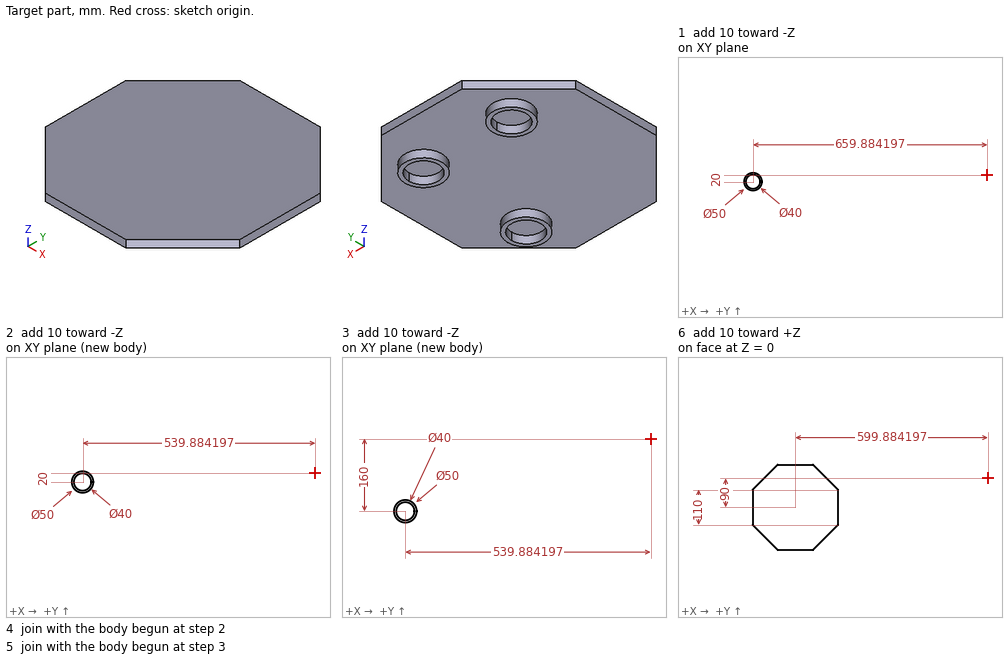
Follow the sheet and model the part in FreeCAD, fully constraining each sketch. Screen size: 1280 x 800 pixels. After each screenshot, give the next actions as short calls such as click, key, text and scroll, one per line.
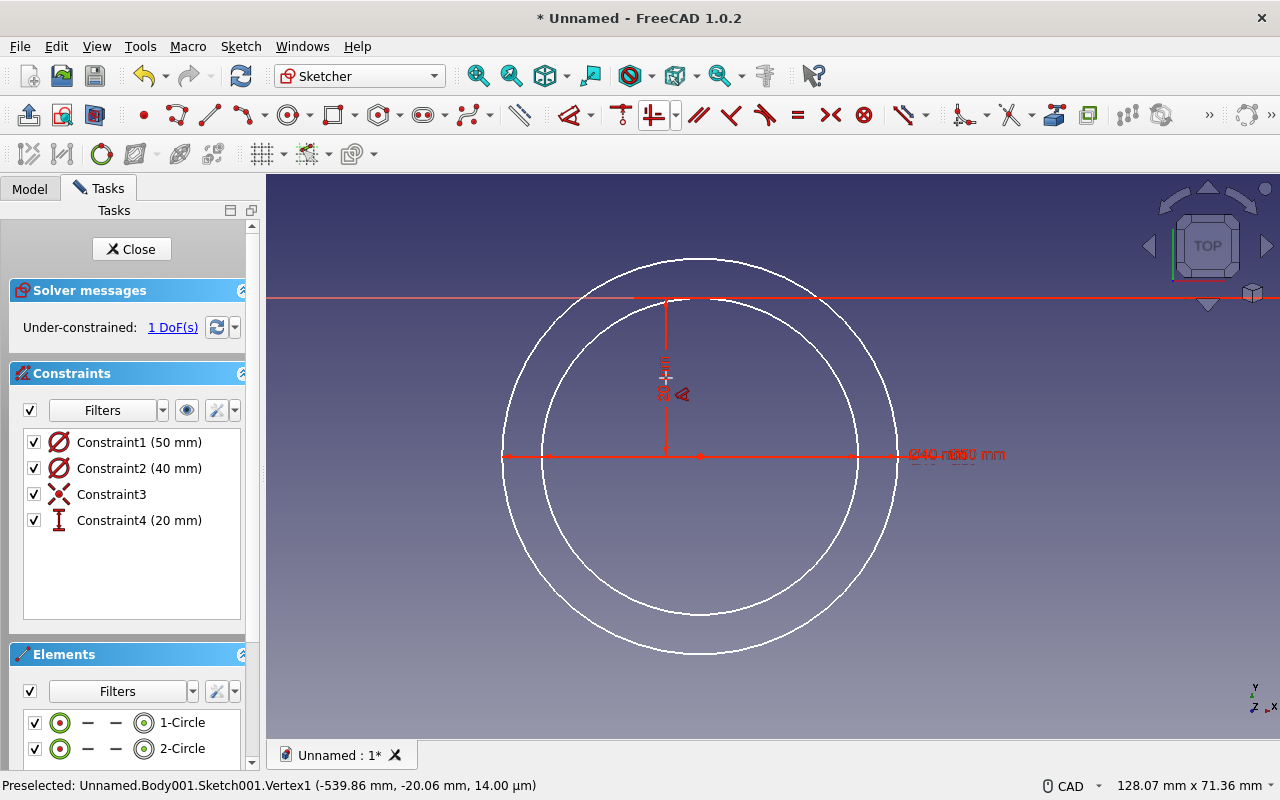
click(700, 456)
click(908, 264)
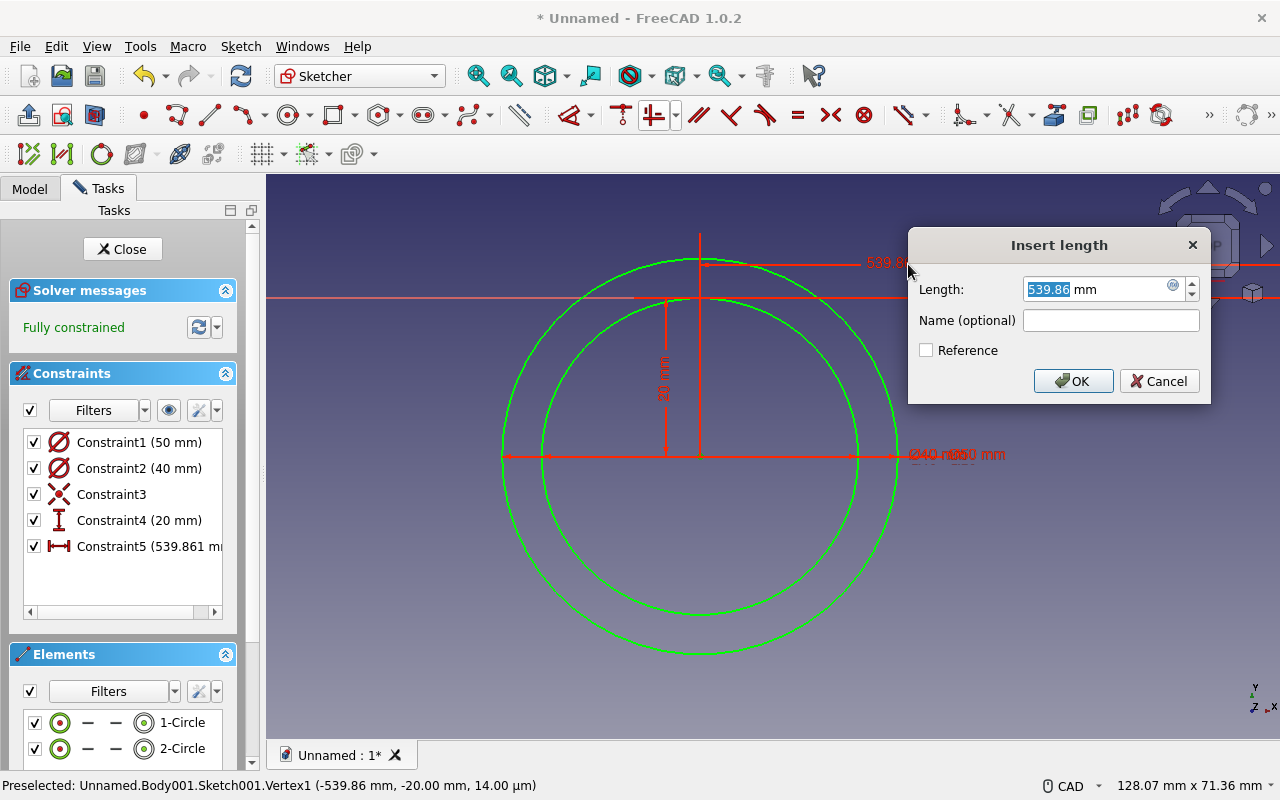
text(539.884197)
key(Return)
key(Escape)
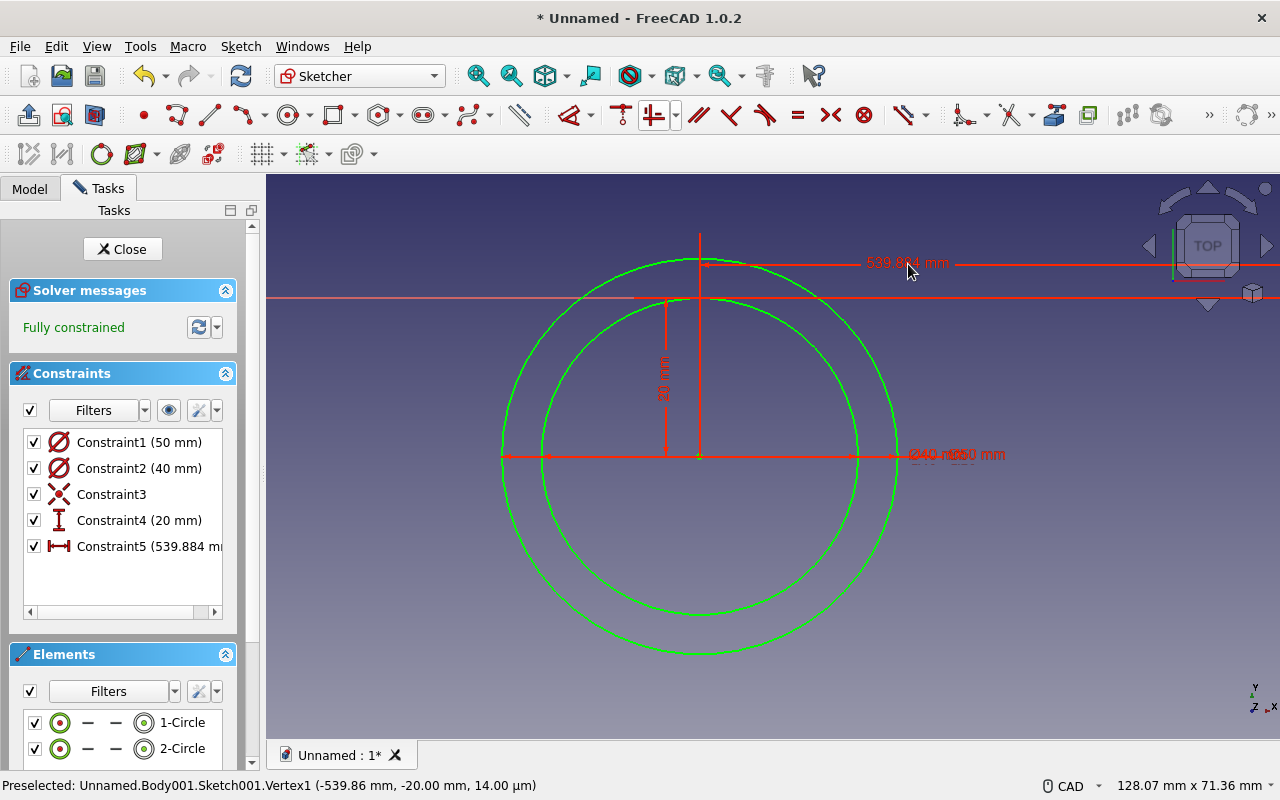
click(123, 249)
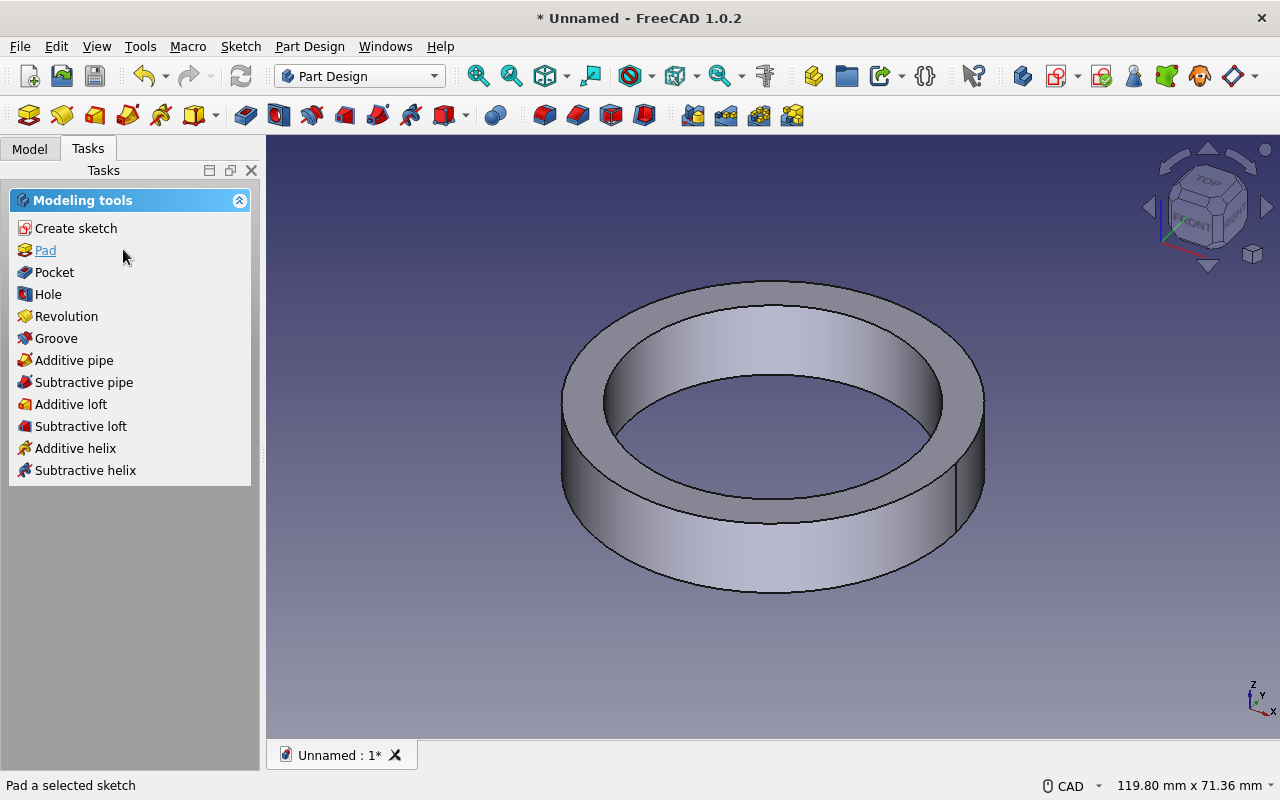
click(29, 116)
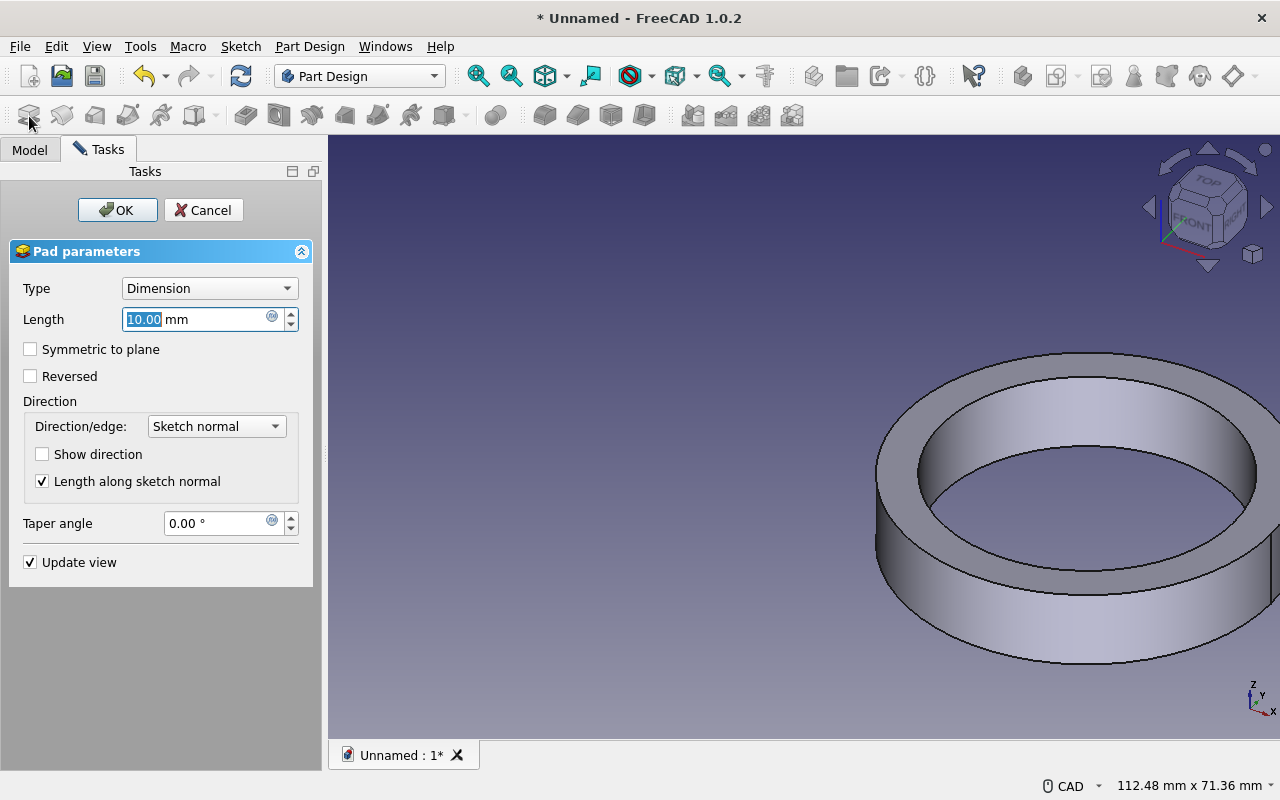
text(10)
key(Tab)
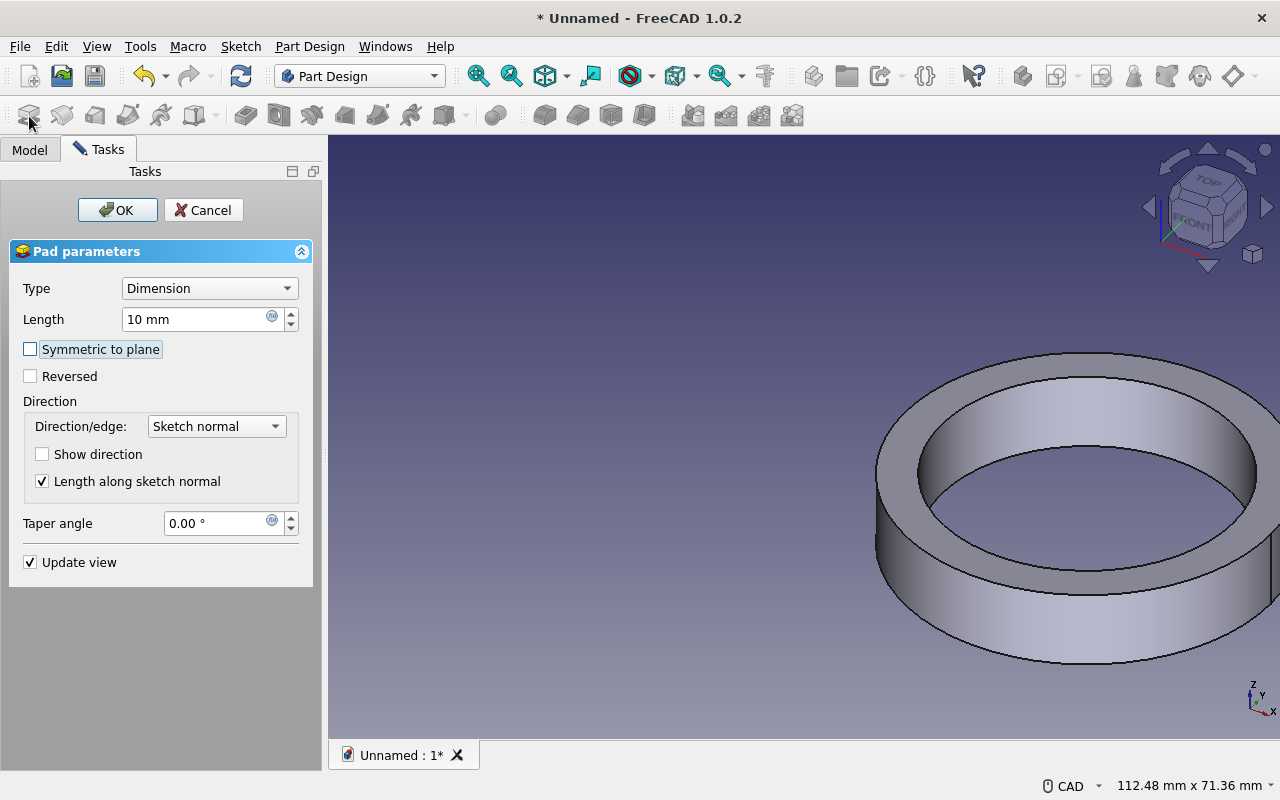
click(31, 376)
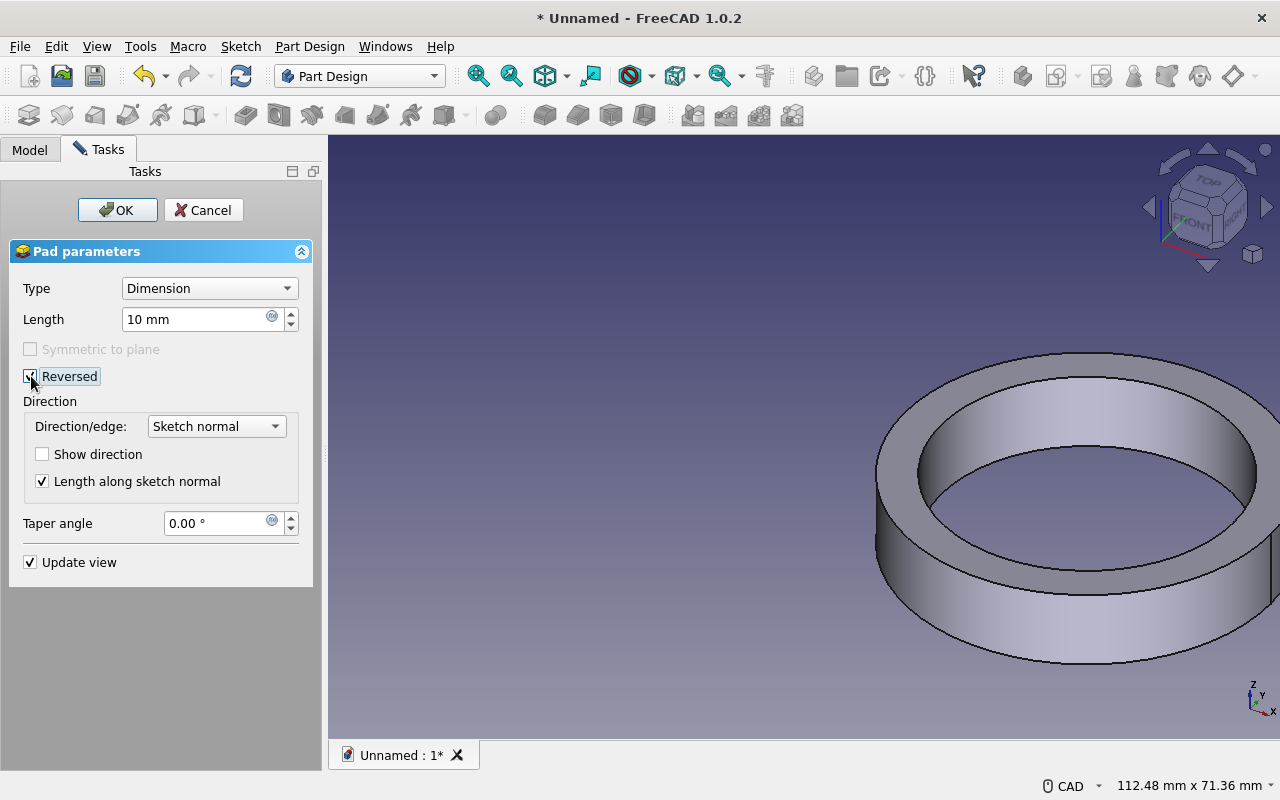
click(118, 210)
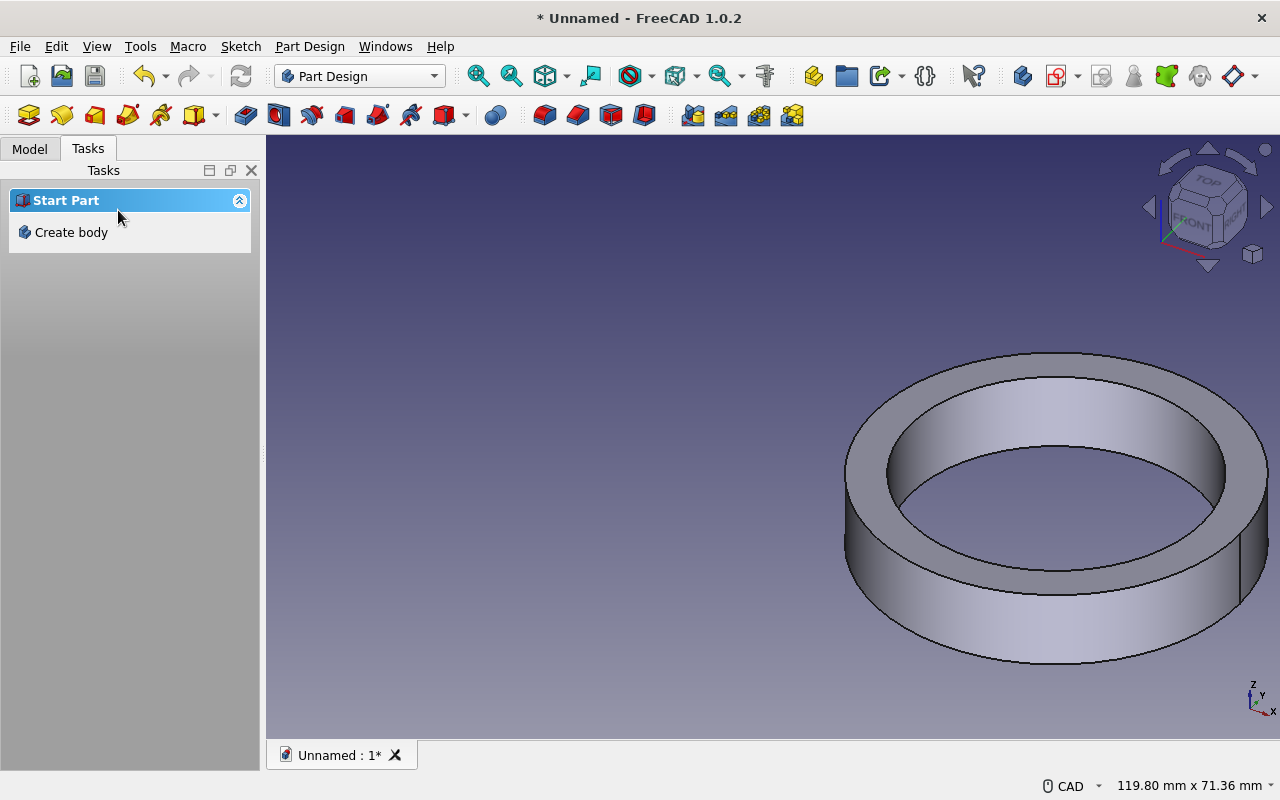
click(479, 76)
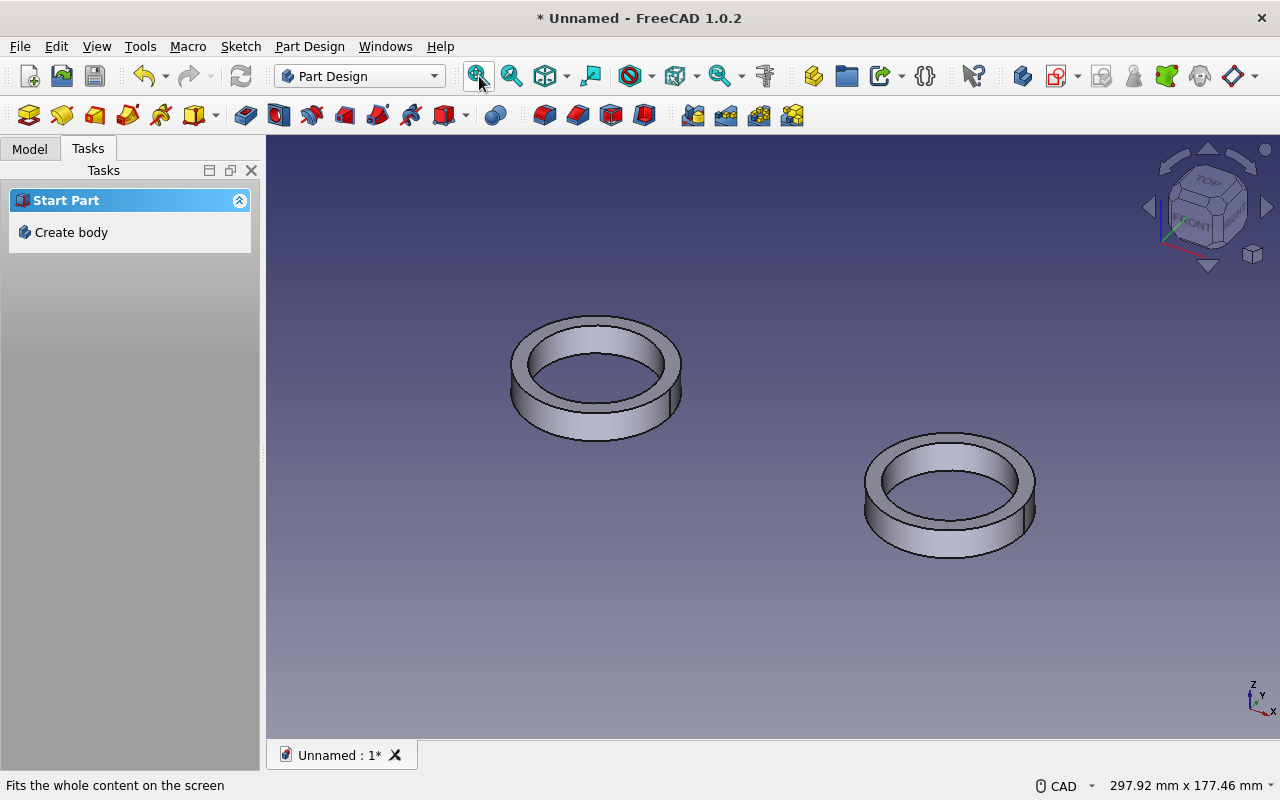
click(1023, 76)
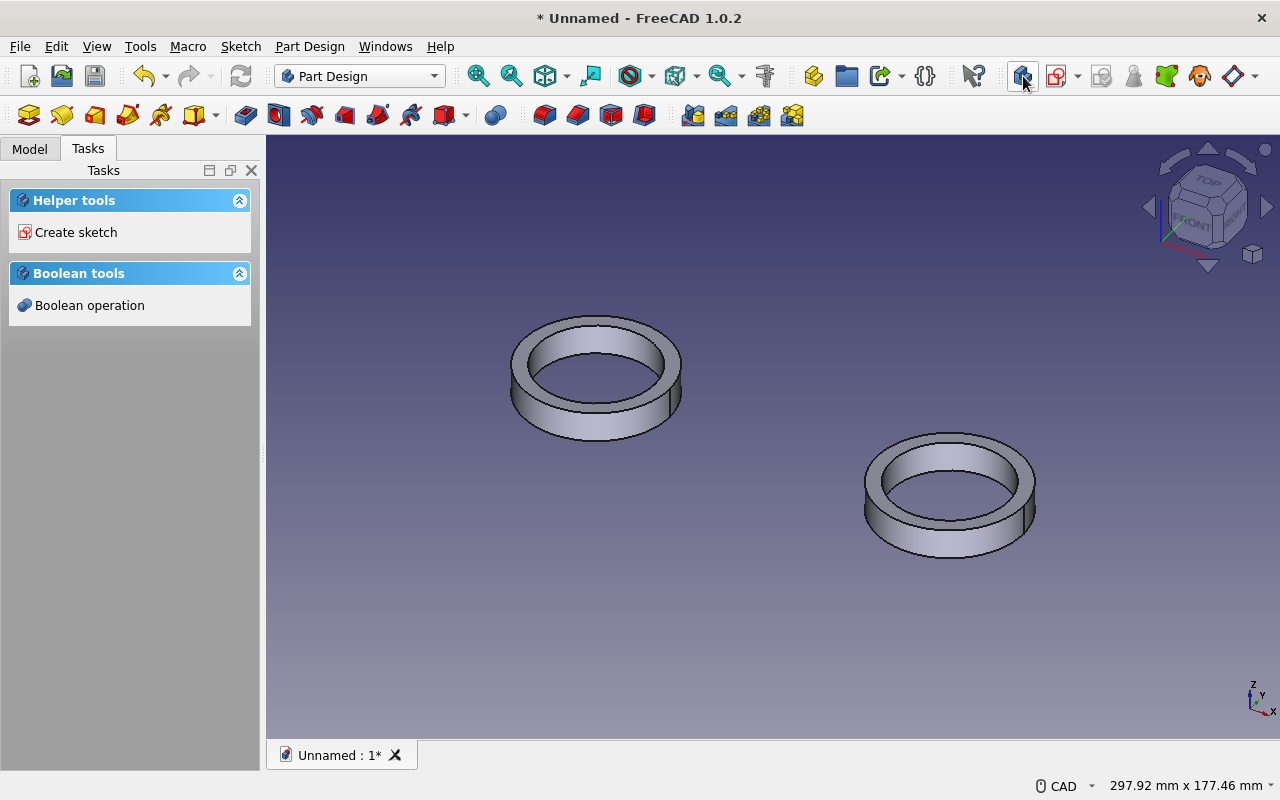
click(306, 699)